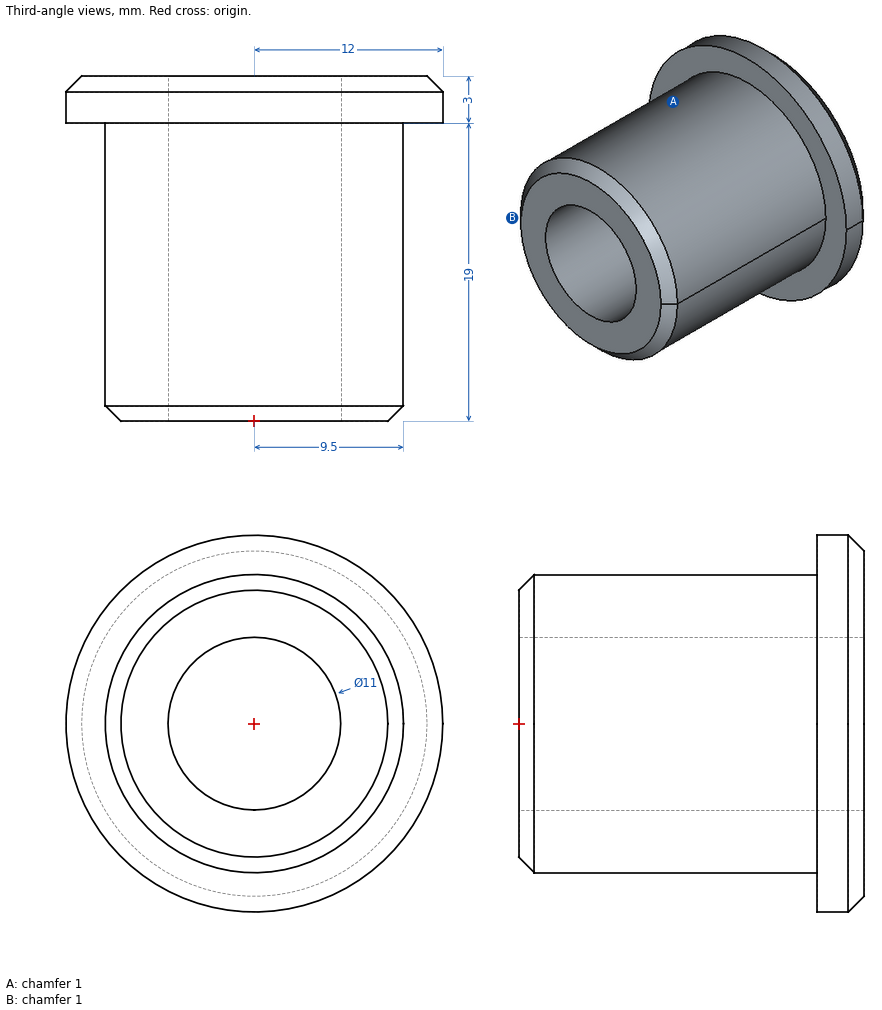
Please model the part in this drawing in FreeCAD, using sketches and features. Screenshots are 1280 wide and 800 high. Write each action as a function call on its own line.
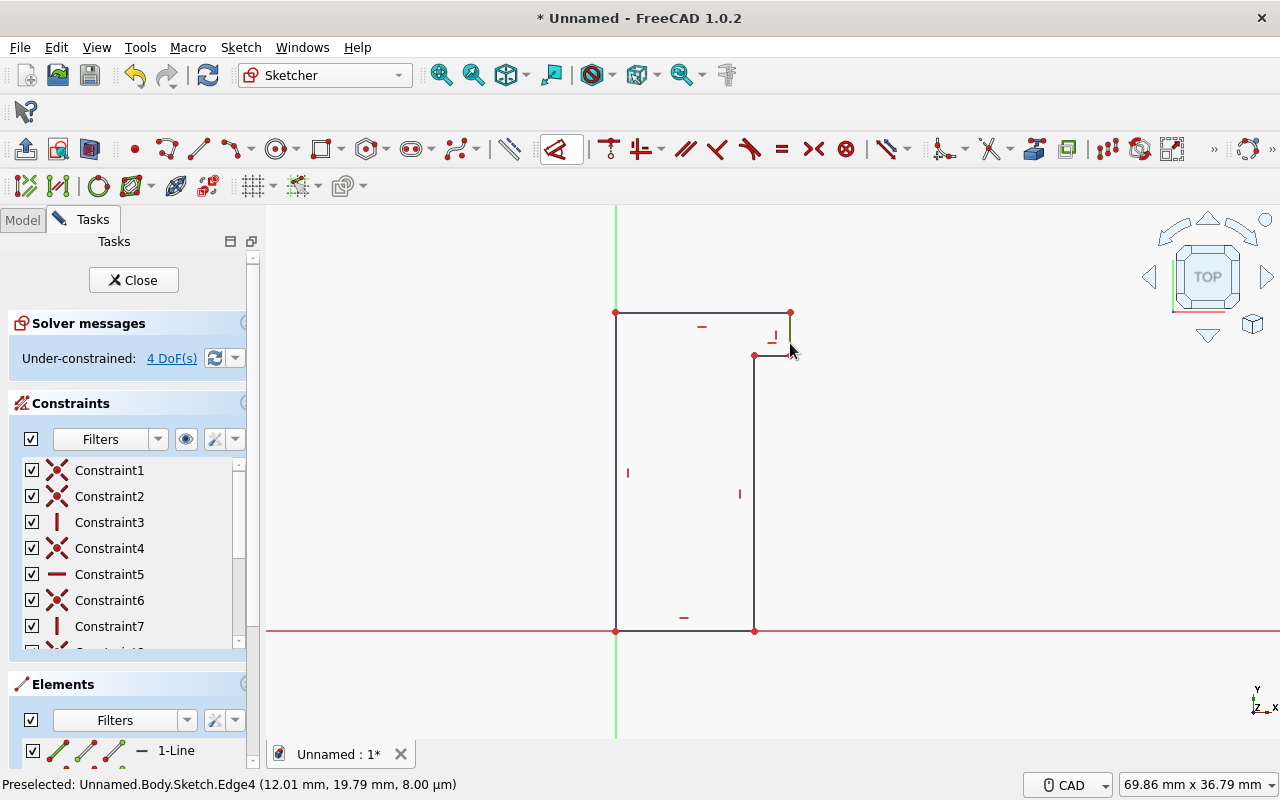
key(i)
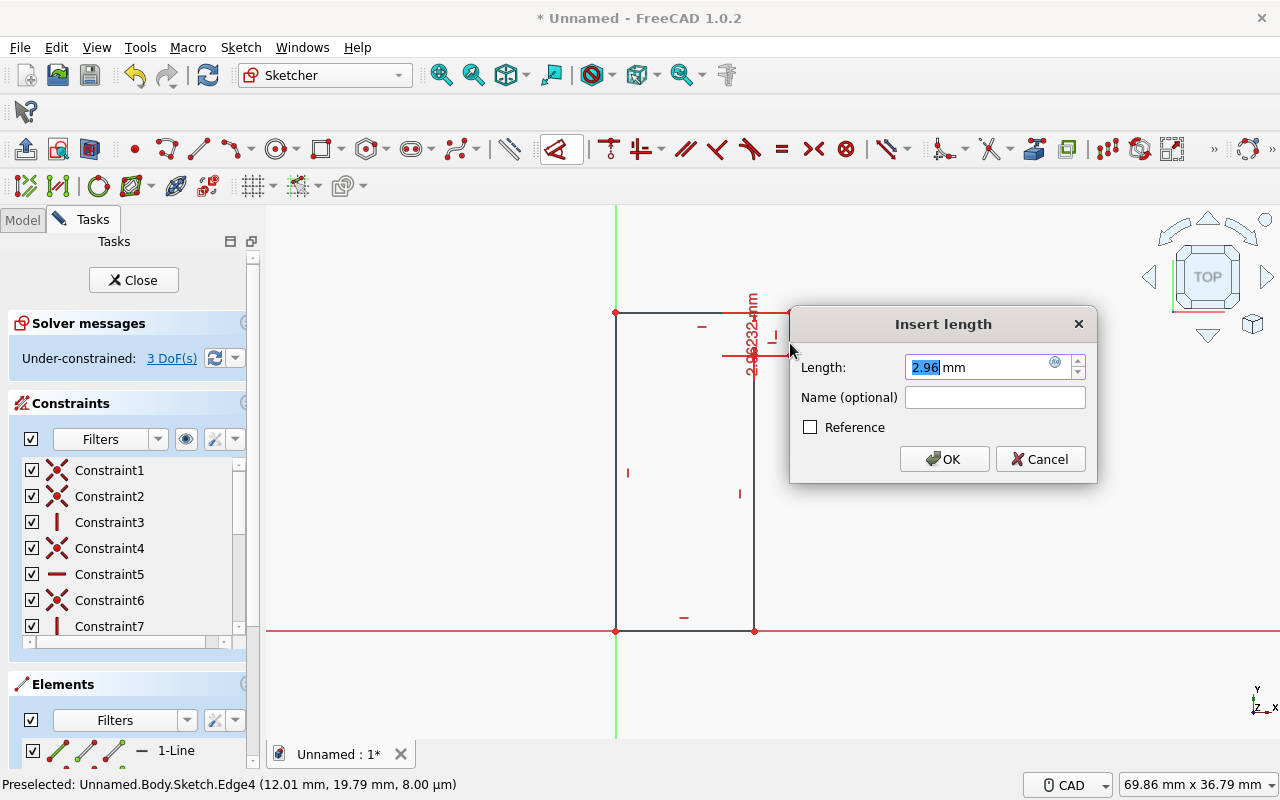
text(3)
key(Return)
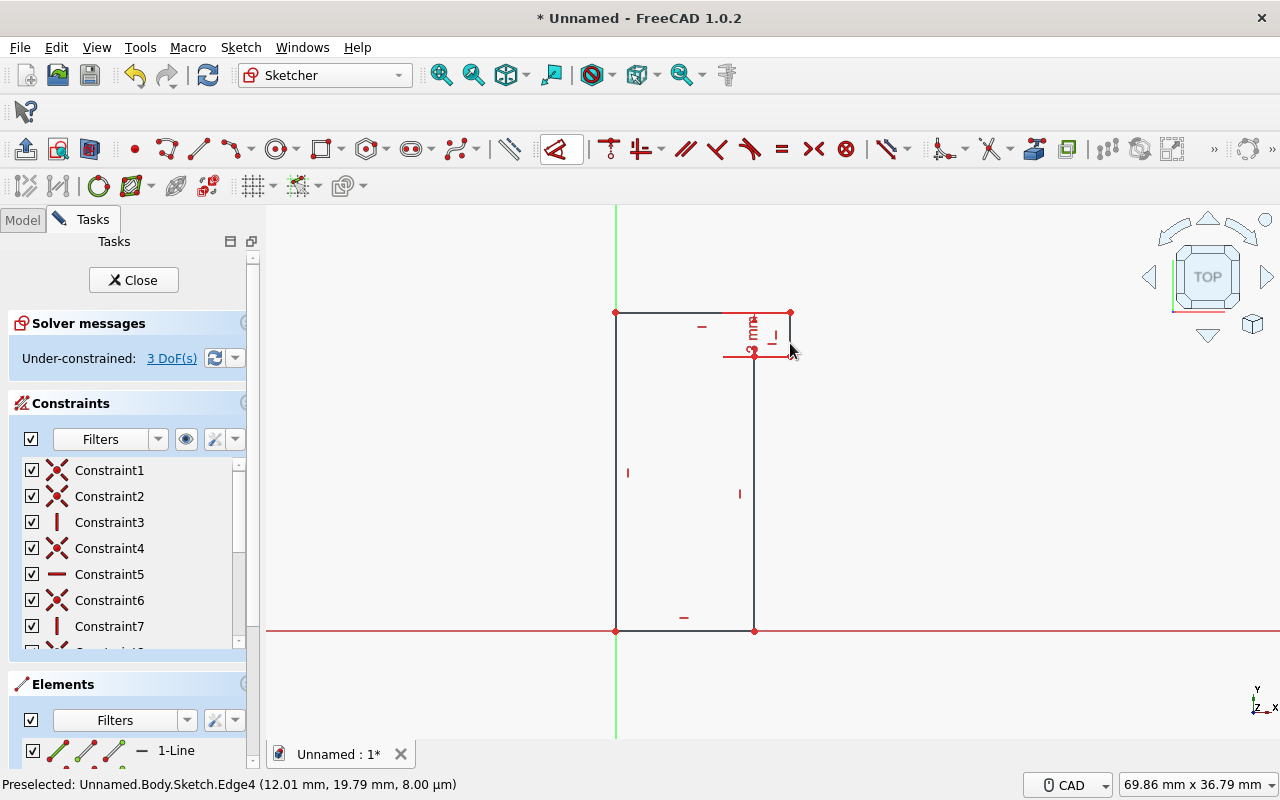
click(754, 549)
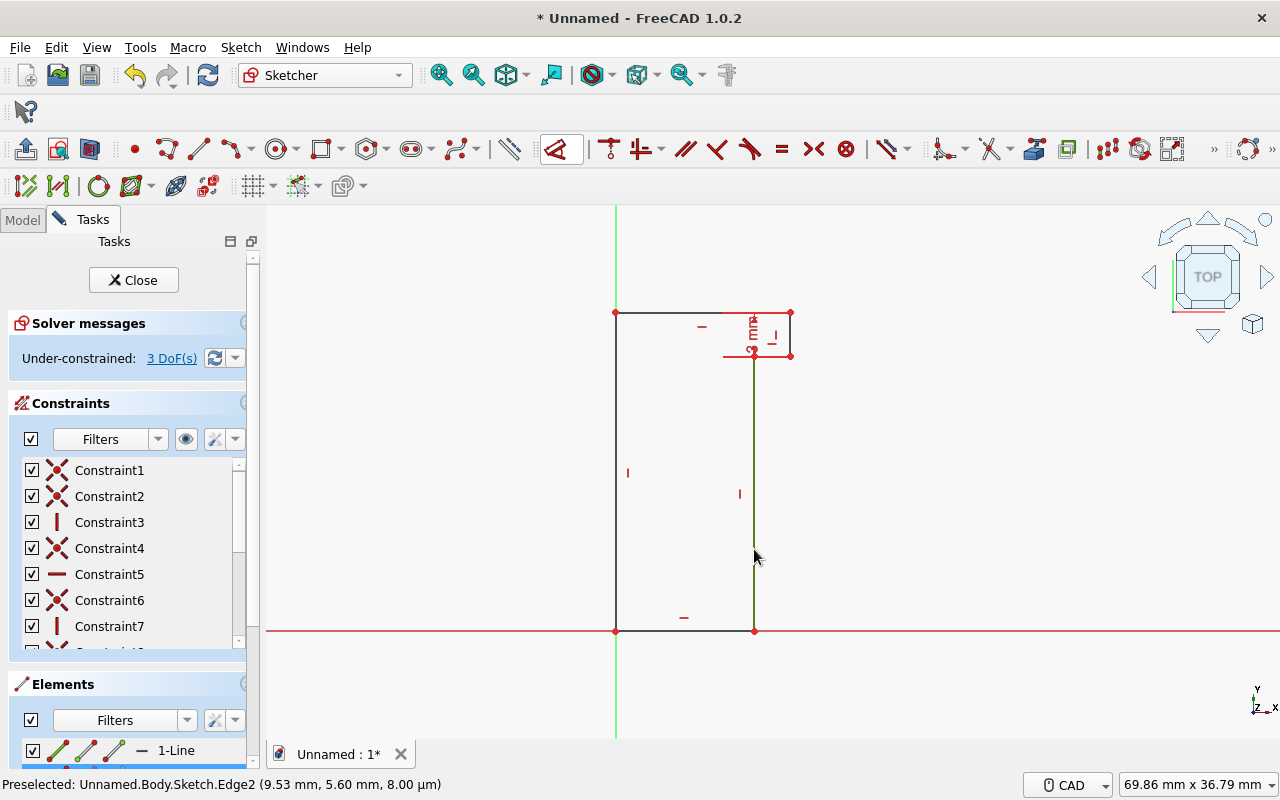
key(i)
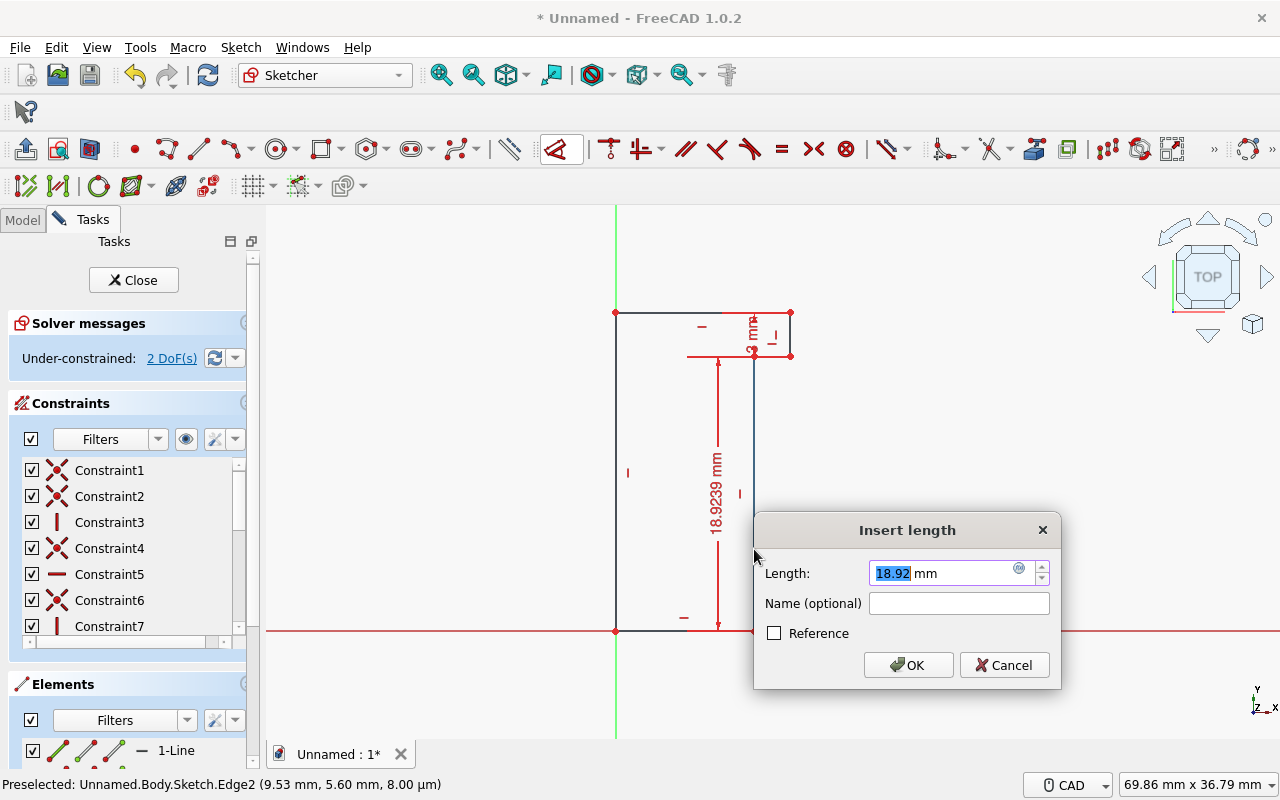
text(19)
key(Return)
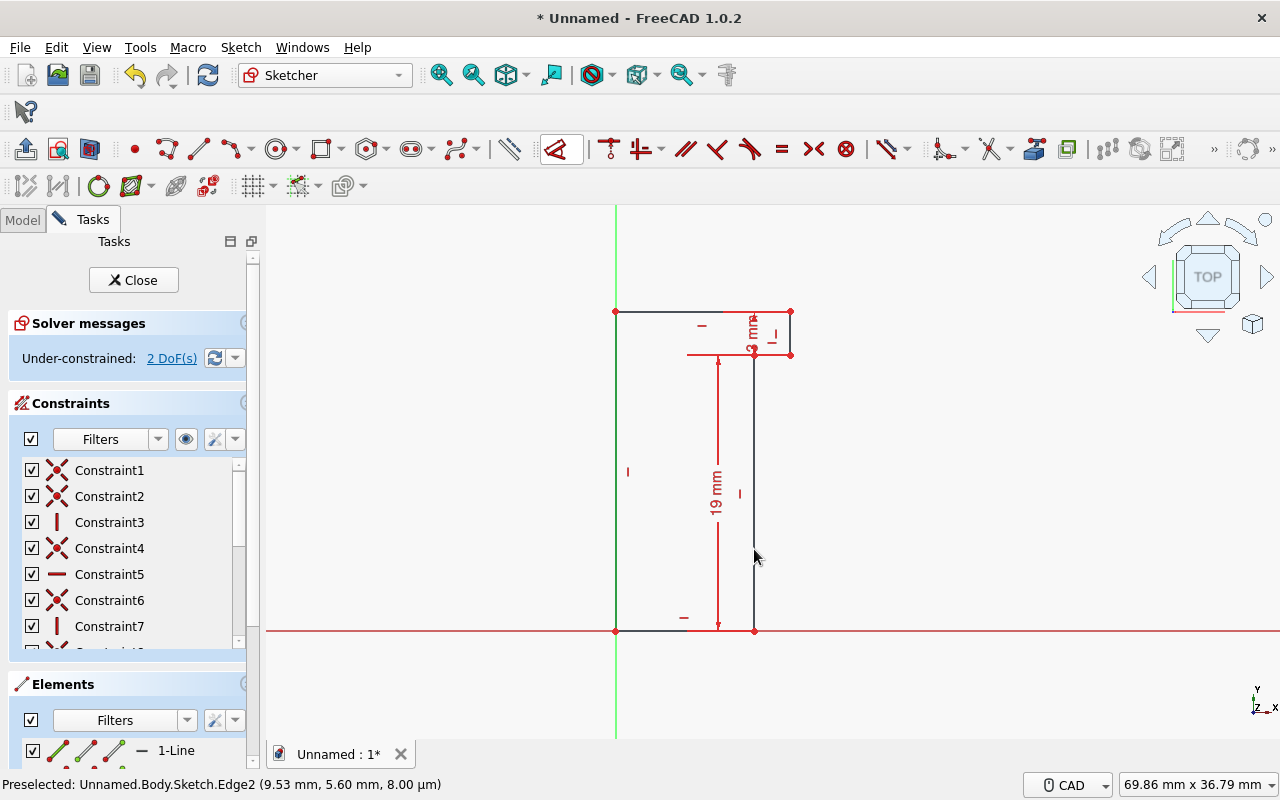
click(738, 312)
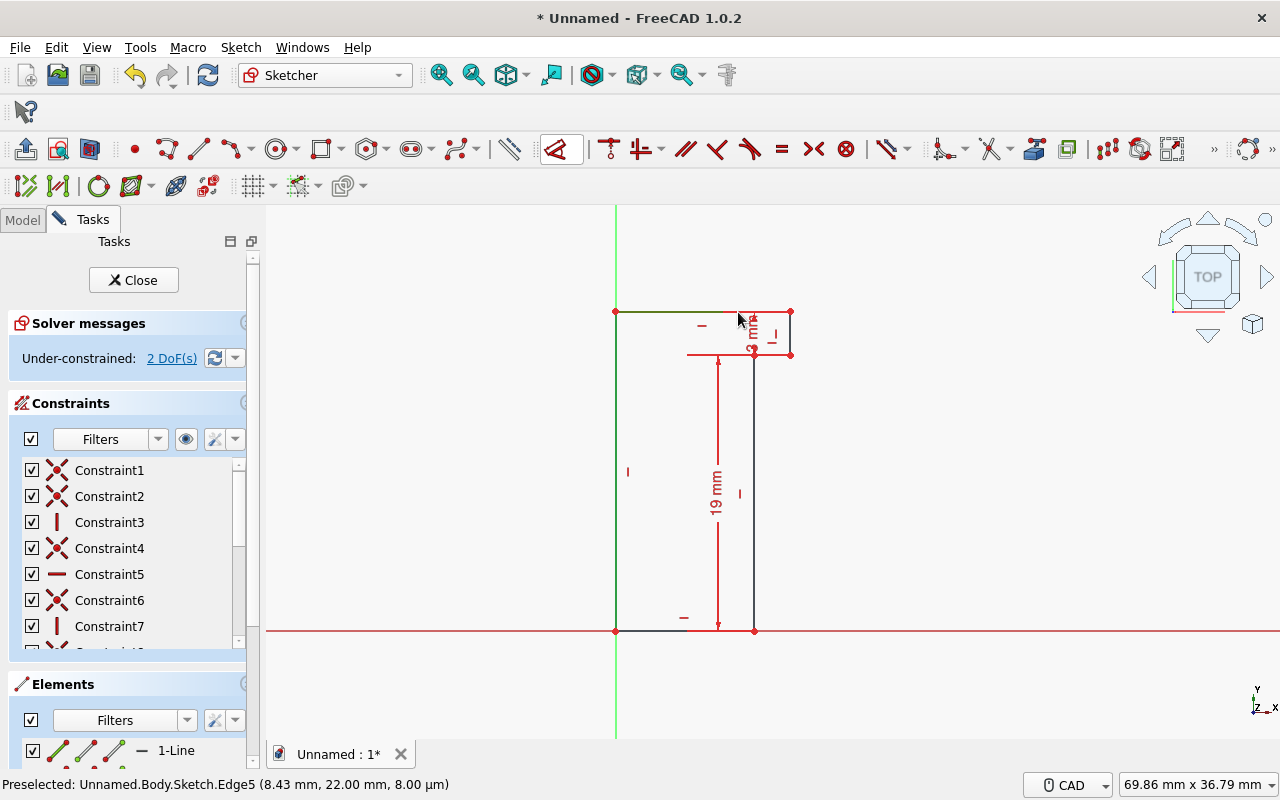
key(l)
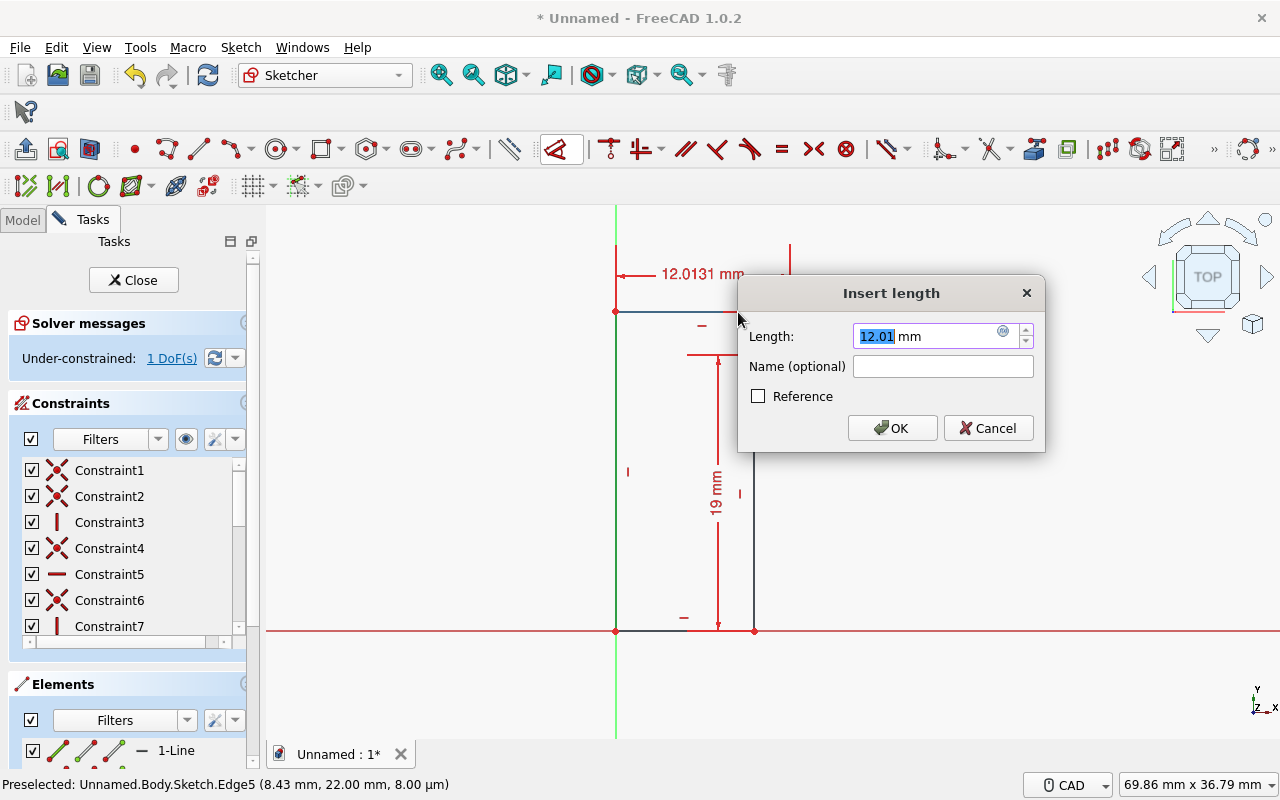
text(12)
key(Return)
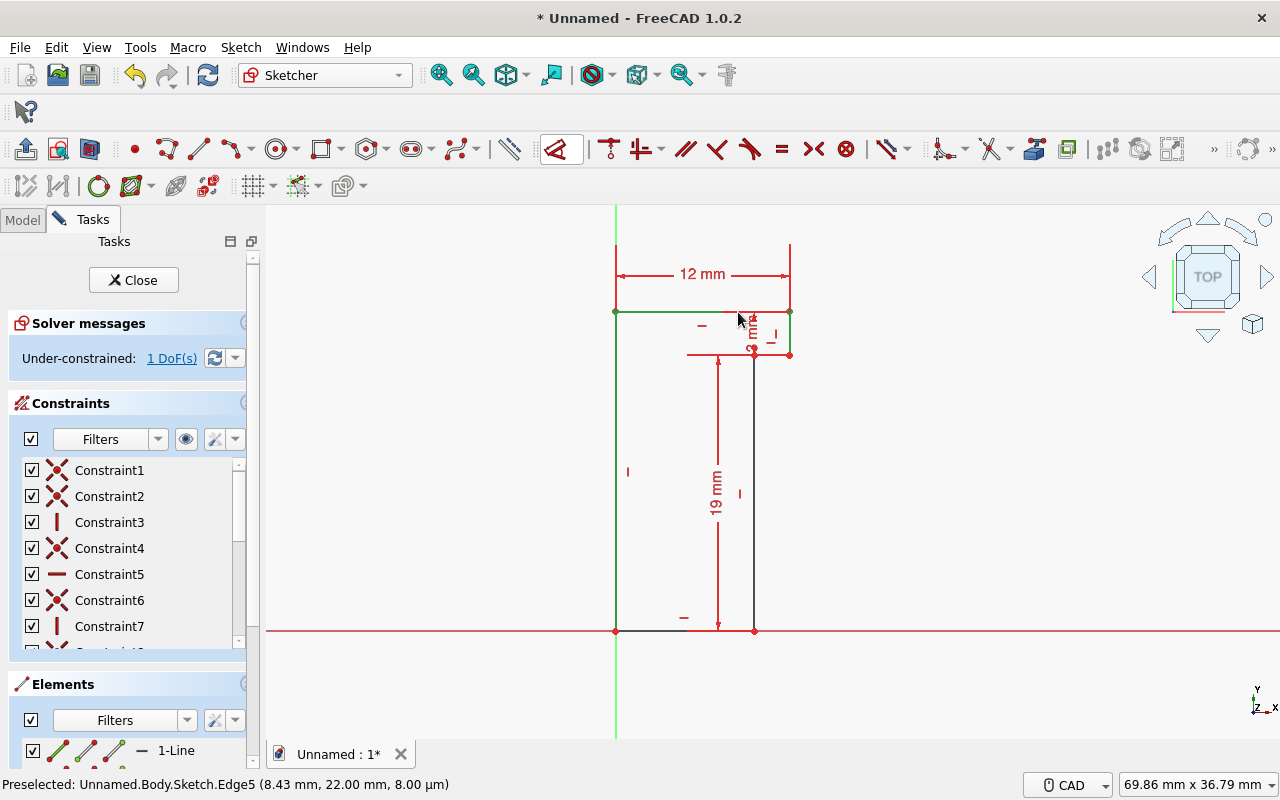
click(657, 631)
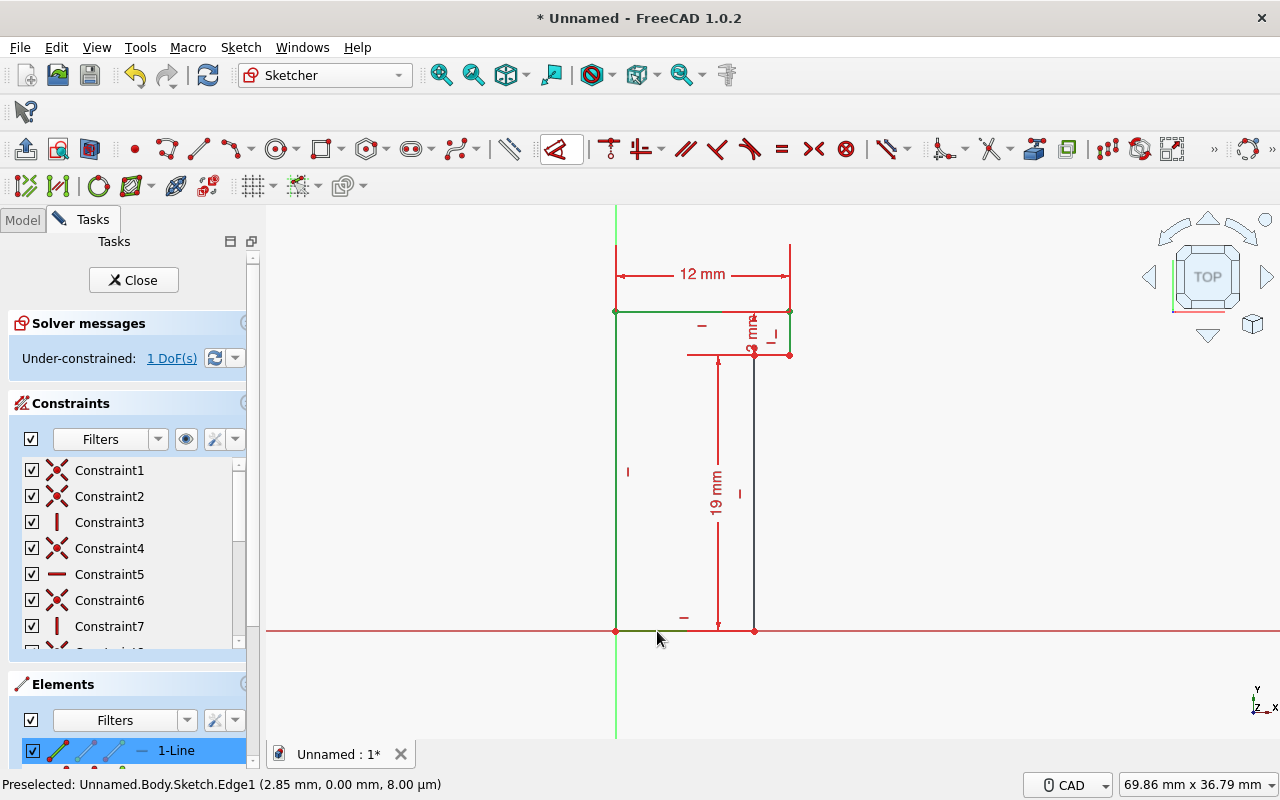
click(578, 150)